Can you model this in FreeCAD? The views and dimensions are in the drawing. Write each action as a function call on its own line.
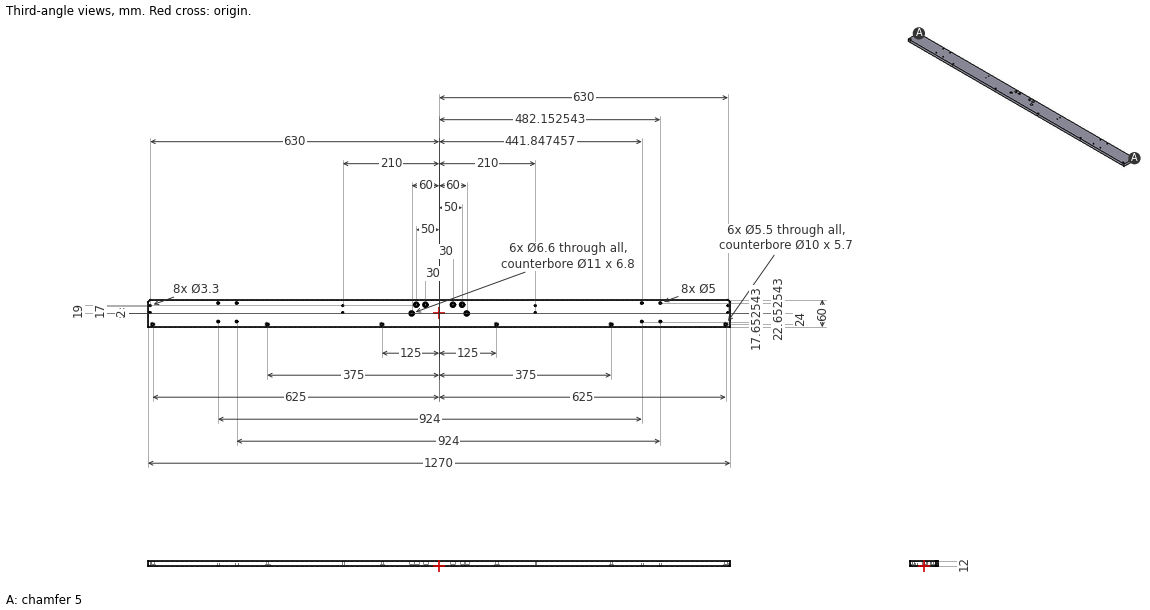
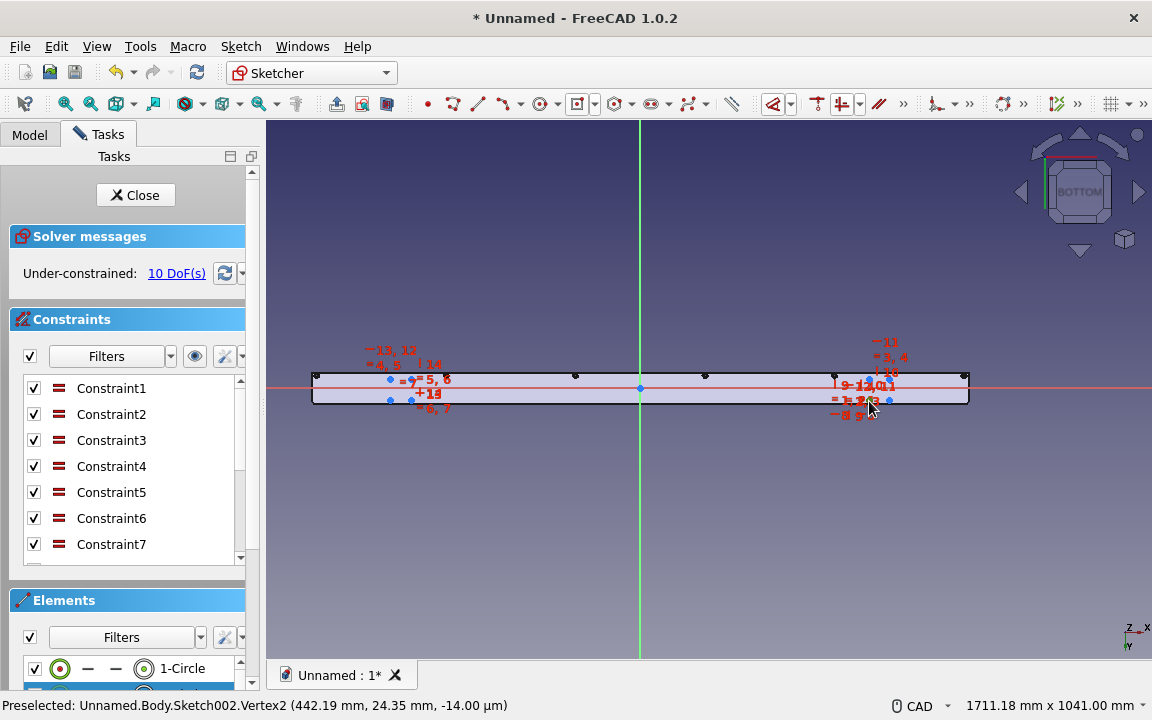
click(411, 401)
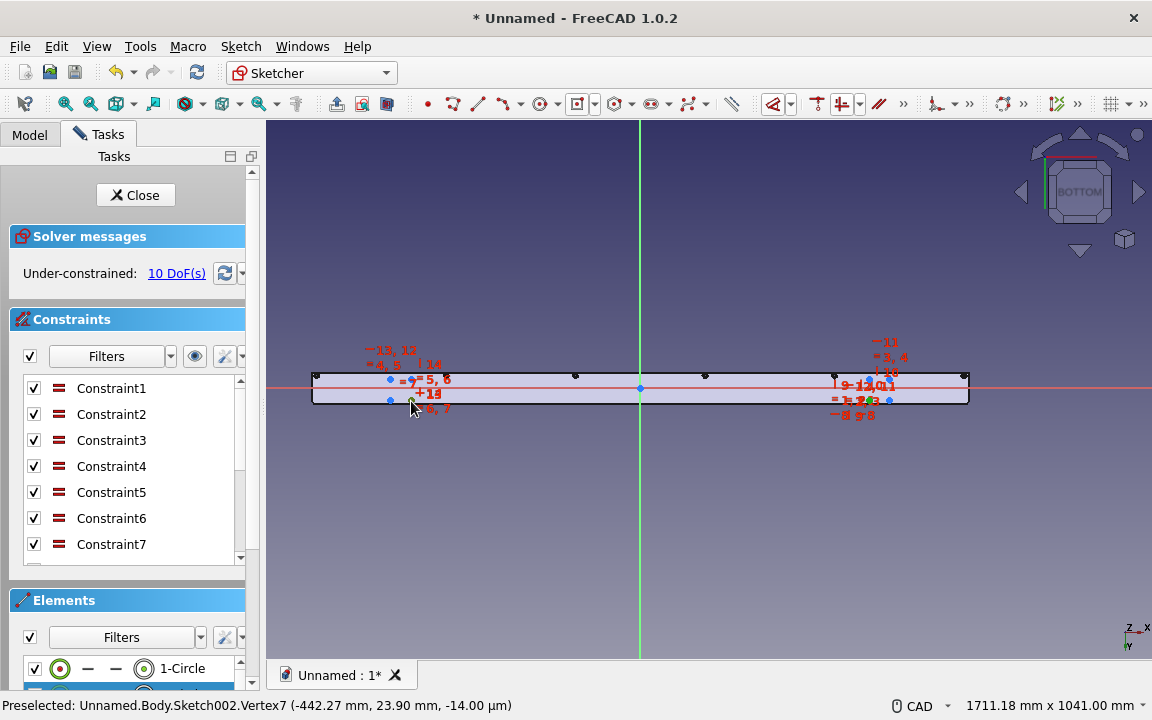
key(h)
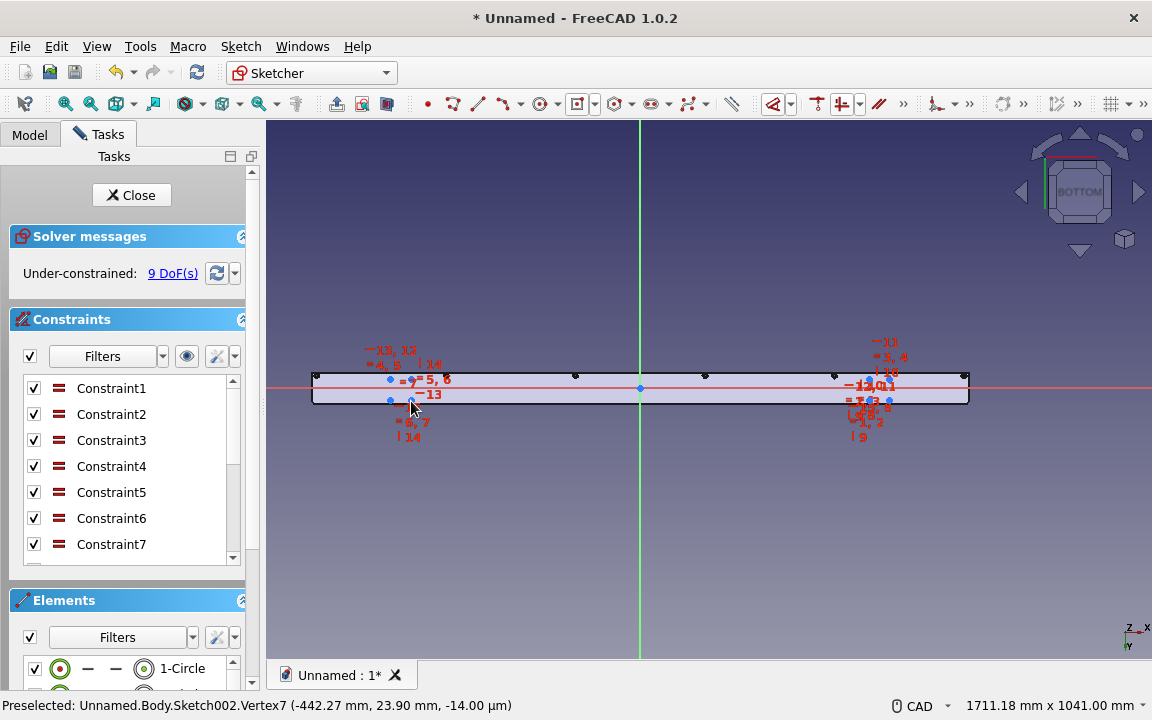
click(391, 380)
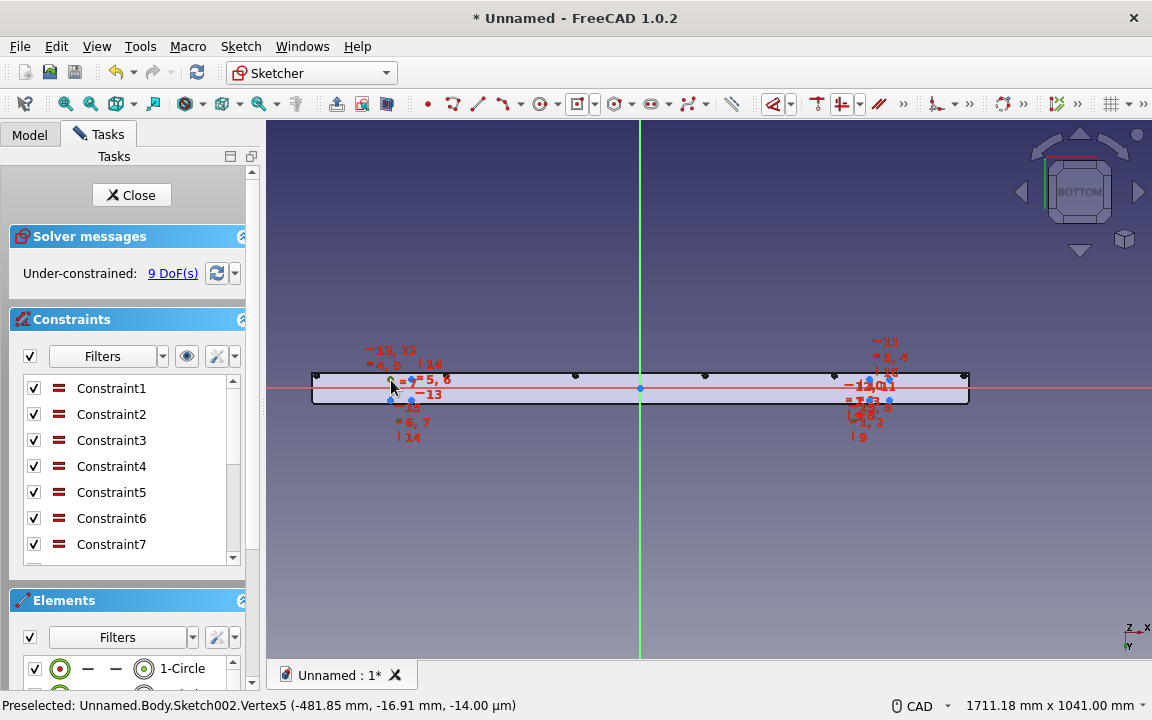
click(391, 400)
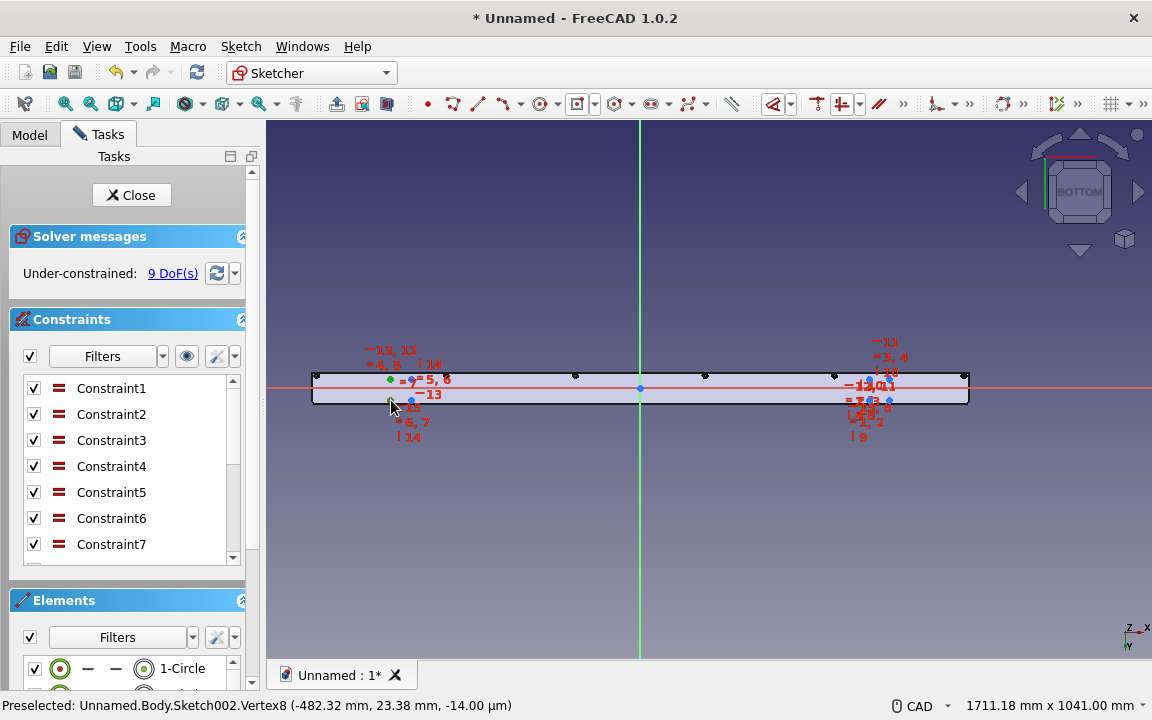
key(v)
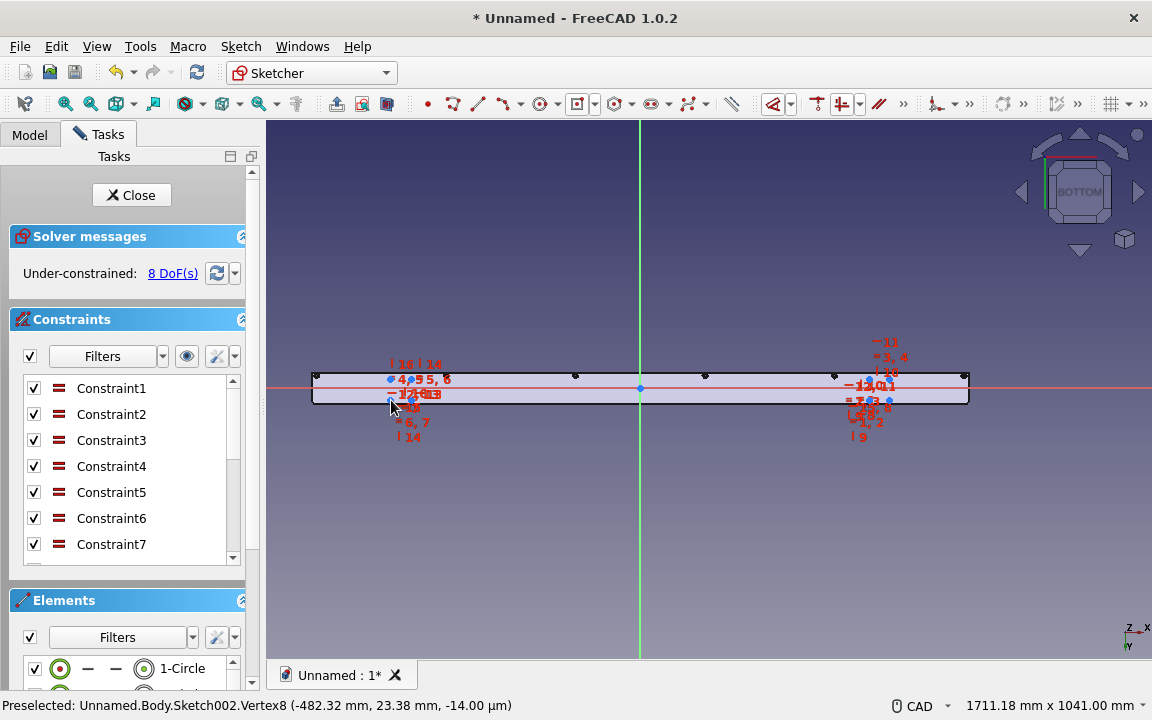
scroll(411, 401, up, 4)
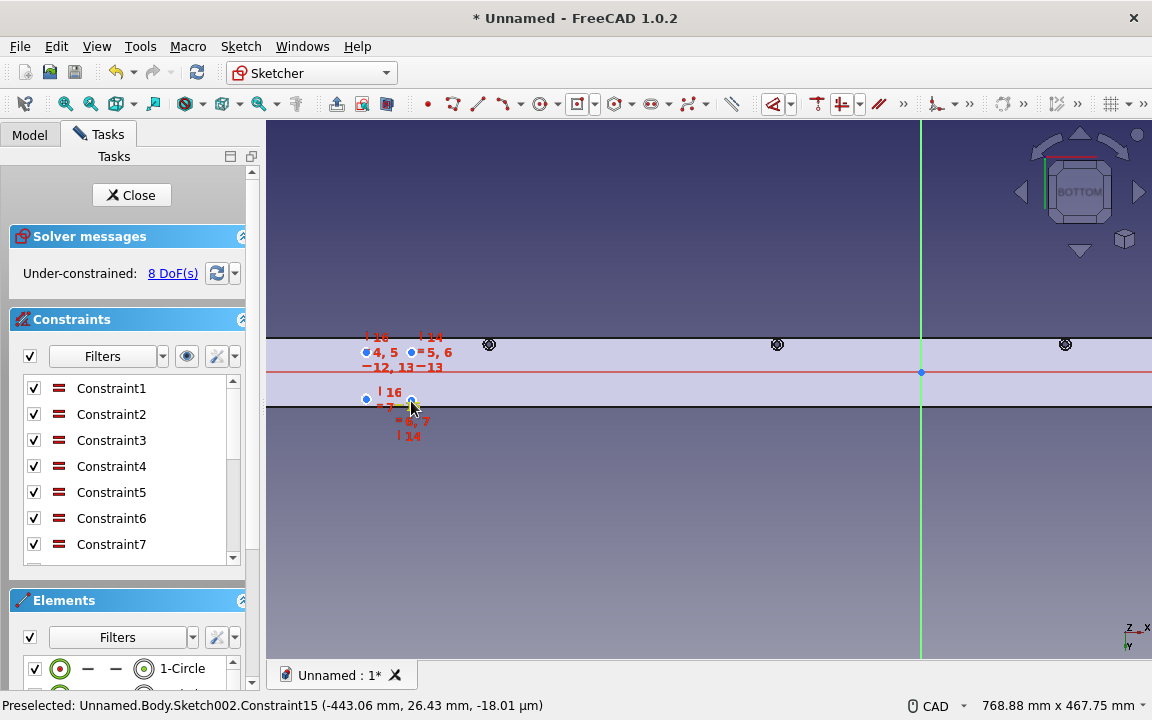
click(410, 398)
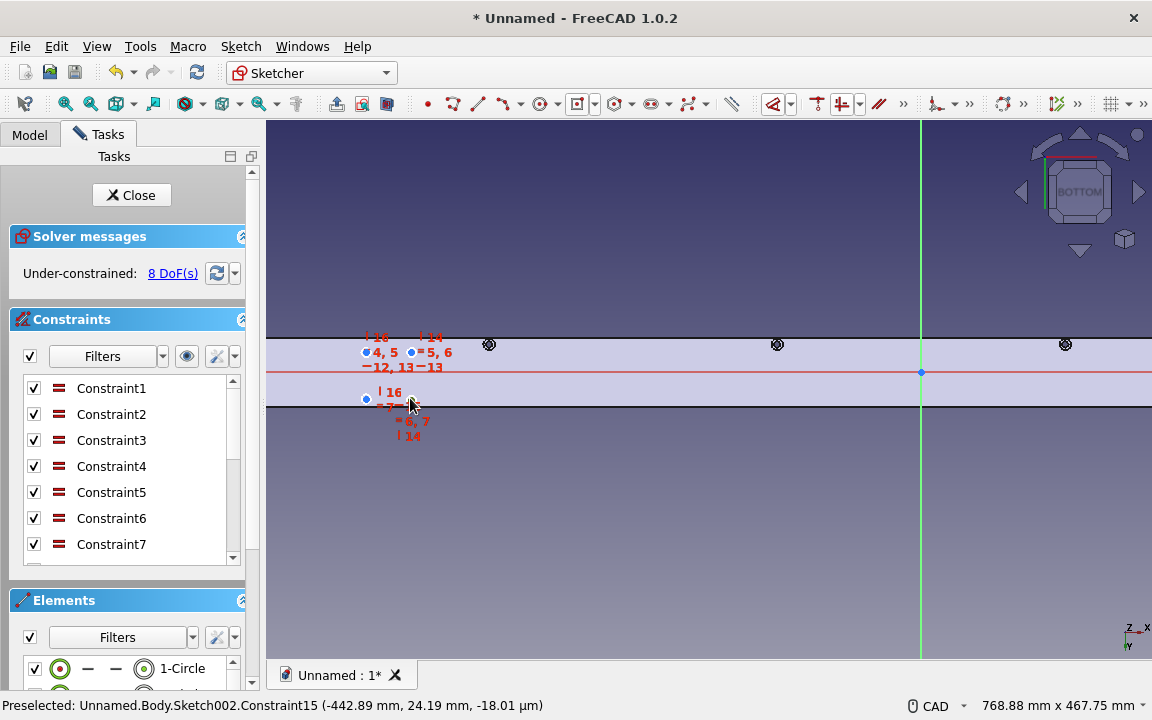
click(366, 399)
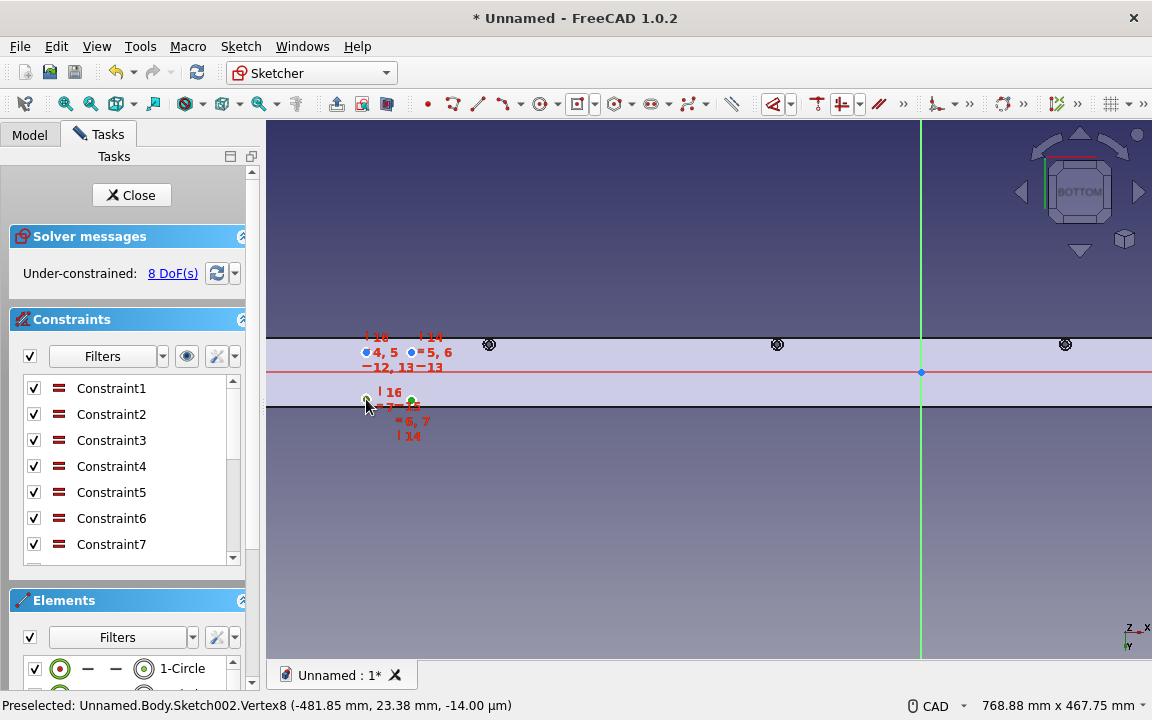
click(860, 104)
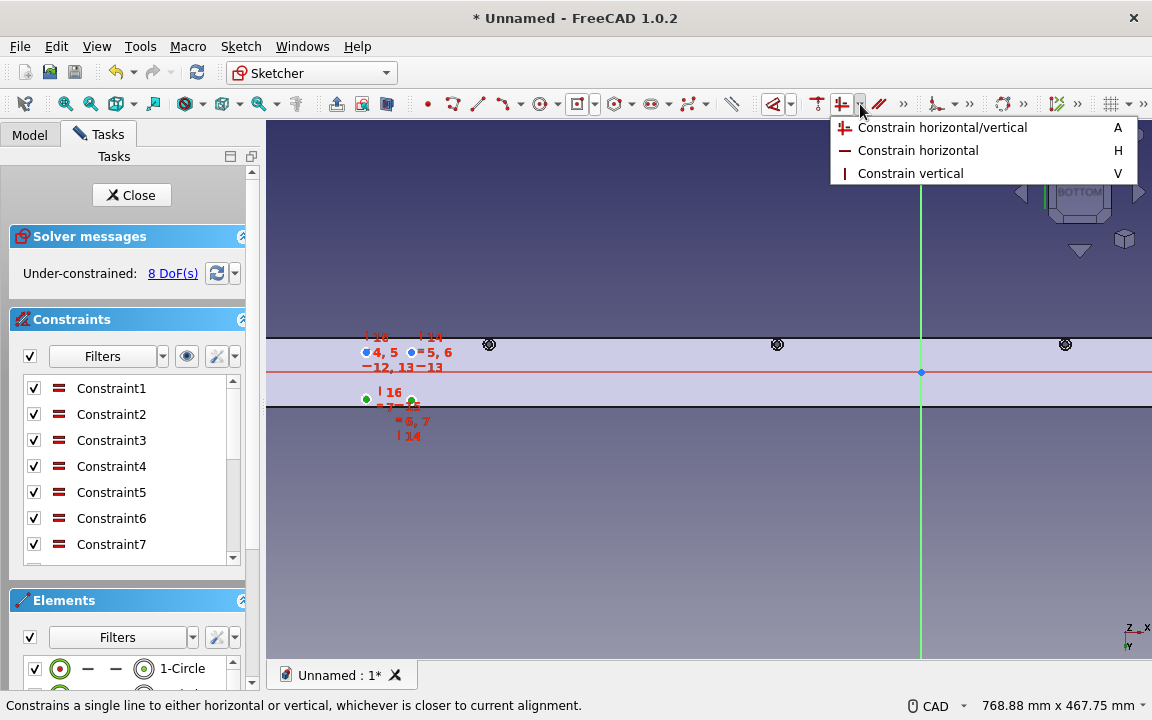
click(984, 150)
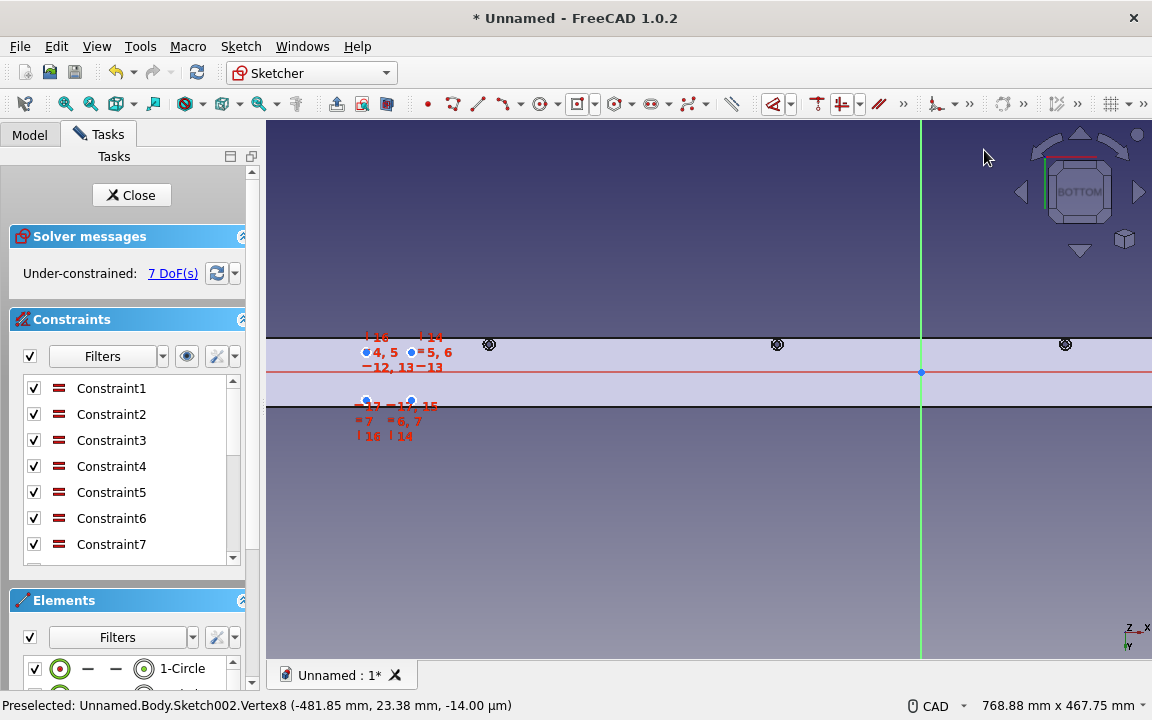
scroll(411, 401, down, 4)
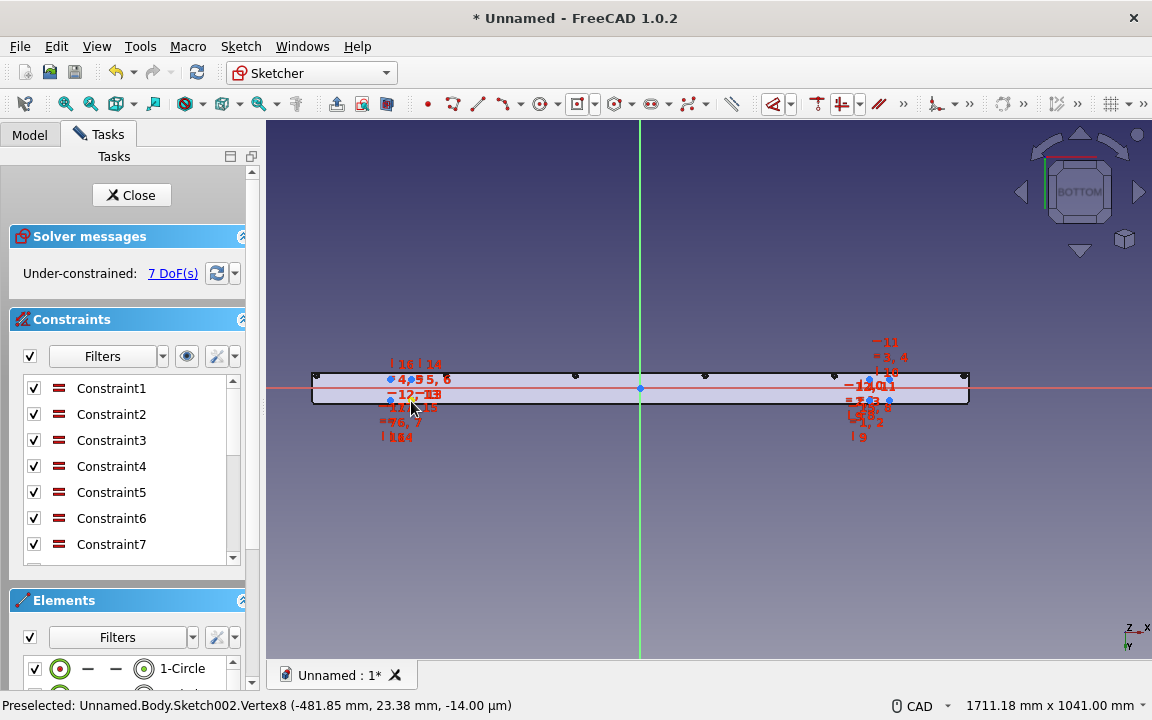
scroll(891, 399, up, 14)